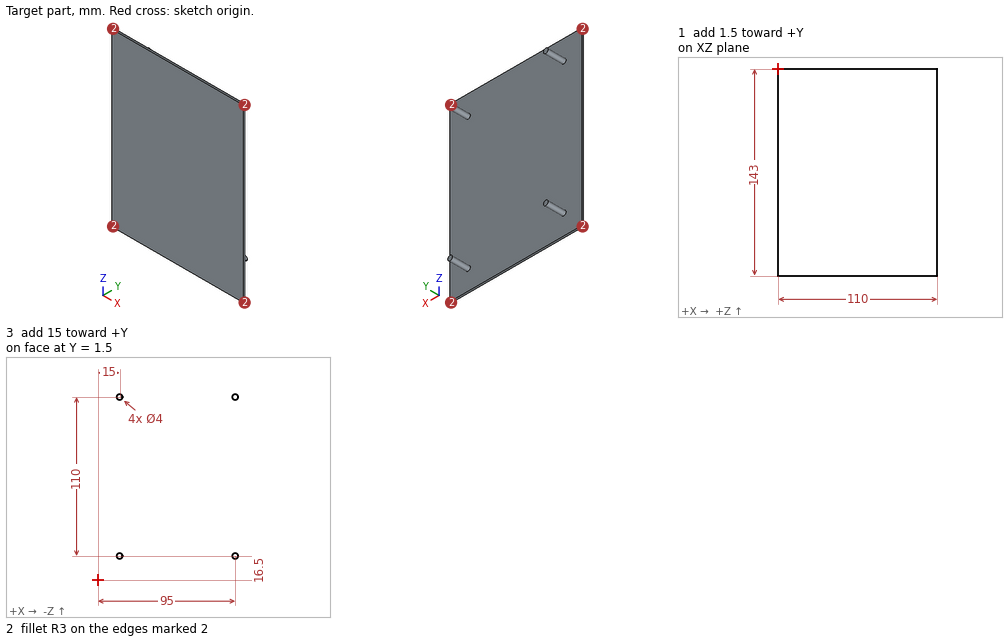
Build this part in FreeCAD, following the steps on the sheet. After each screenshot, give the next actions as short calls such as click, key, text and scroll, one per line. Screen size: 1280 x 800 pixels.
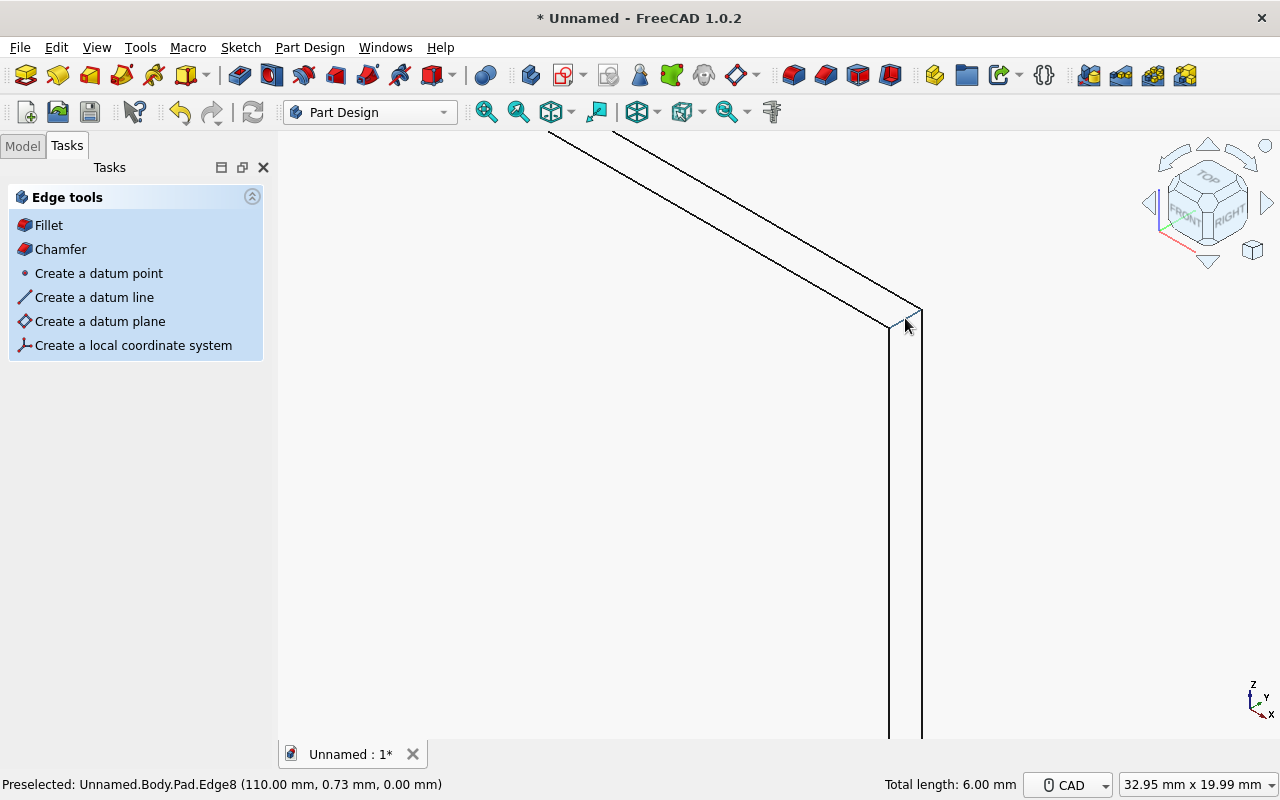
key(v)
key(1)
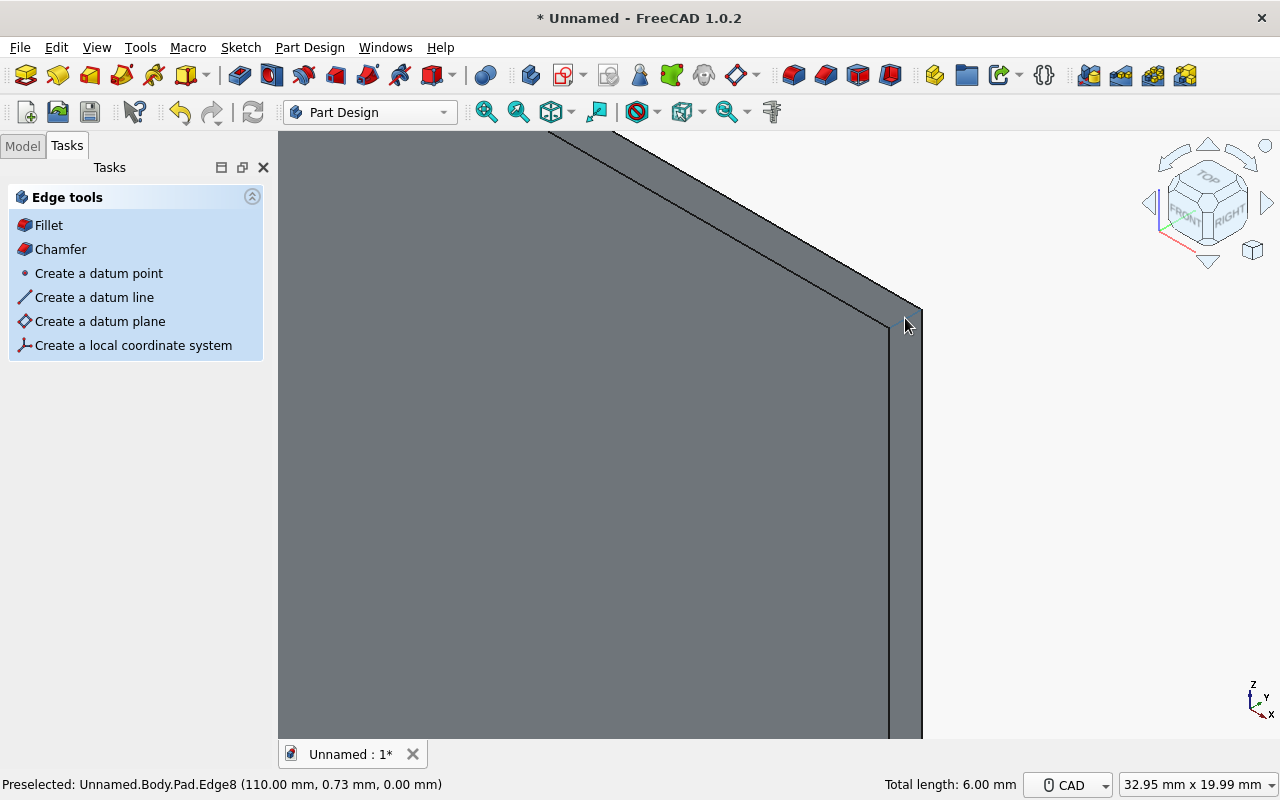
click(794, 76)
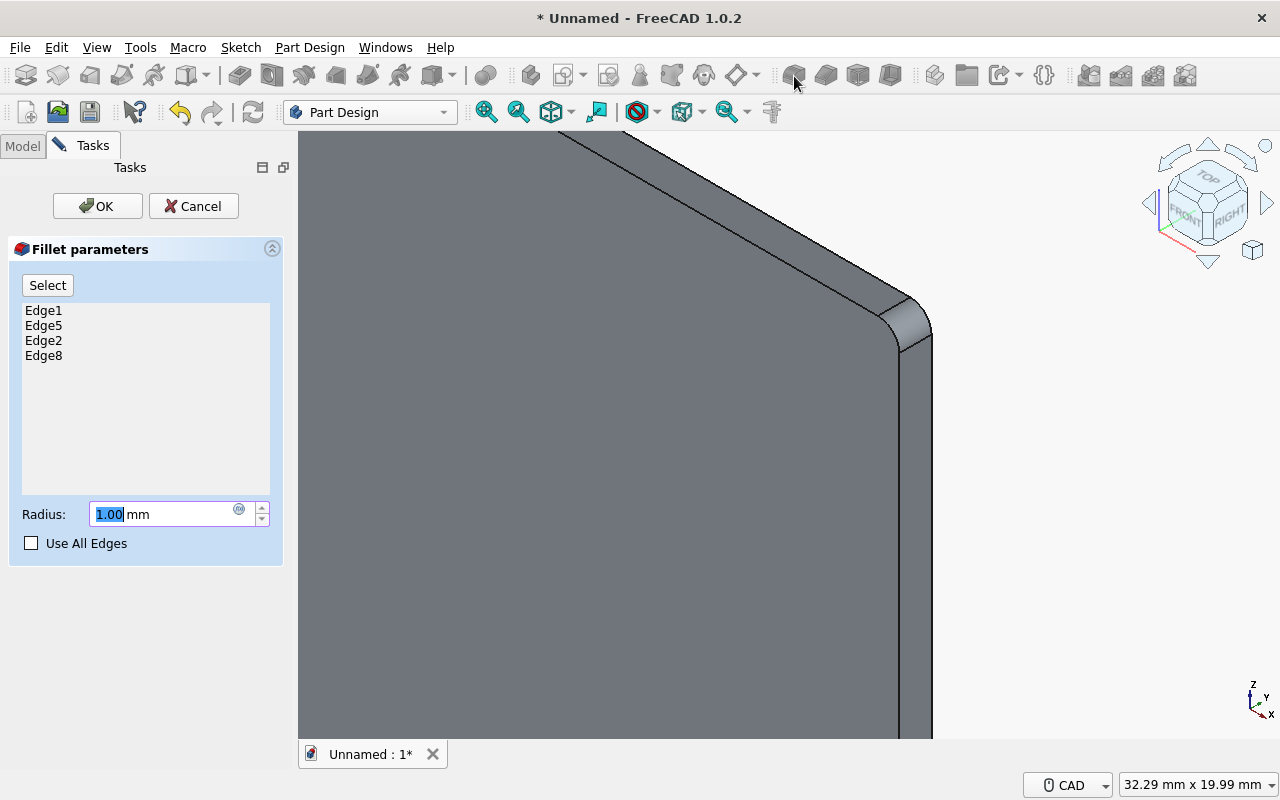
text(3)
key(Tab)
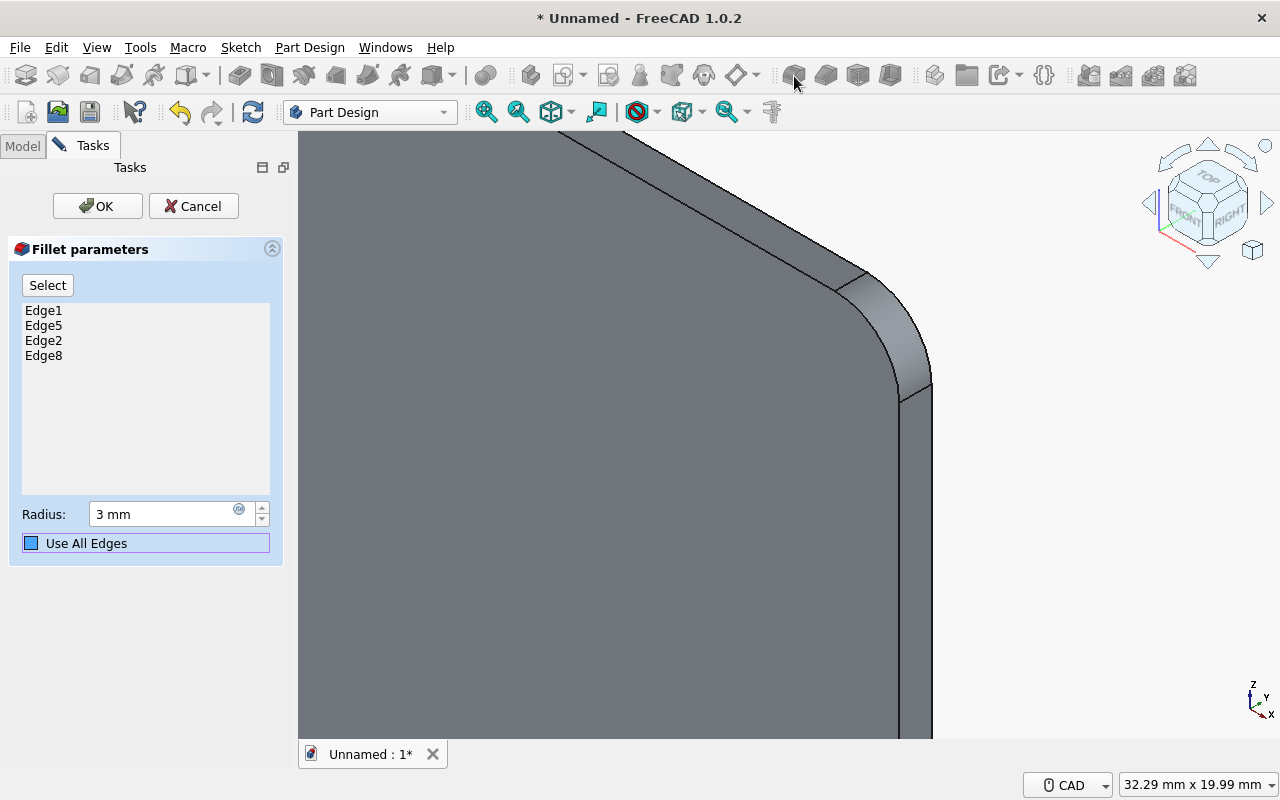
click(98, 206)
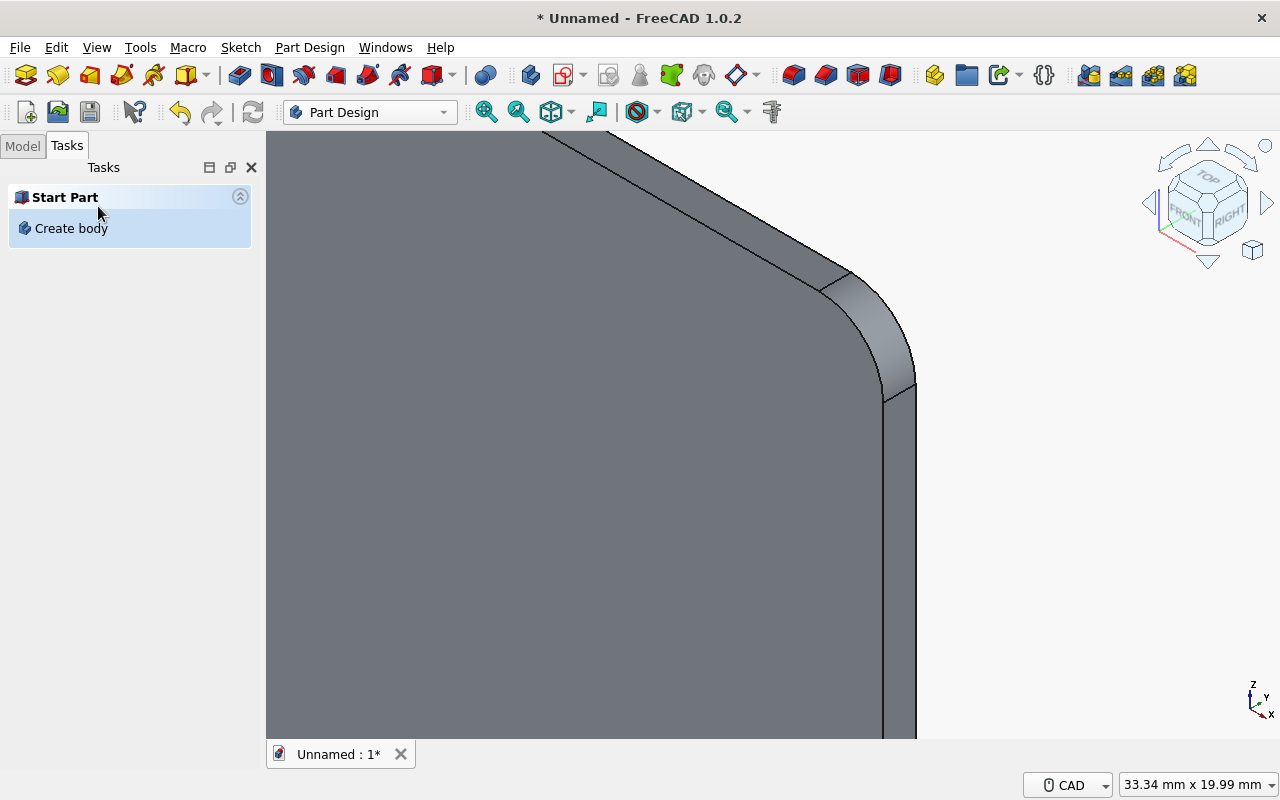
click(488, 112)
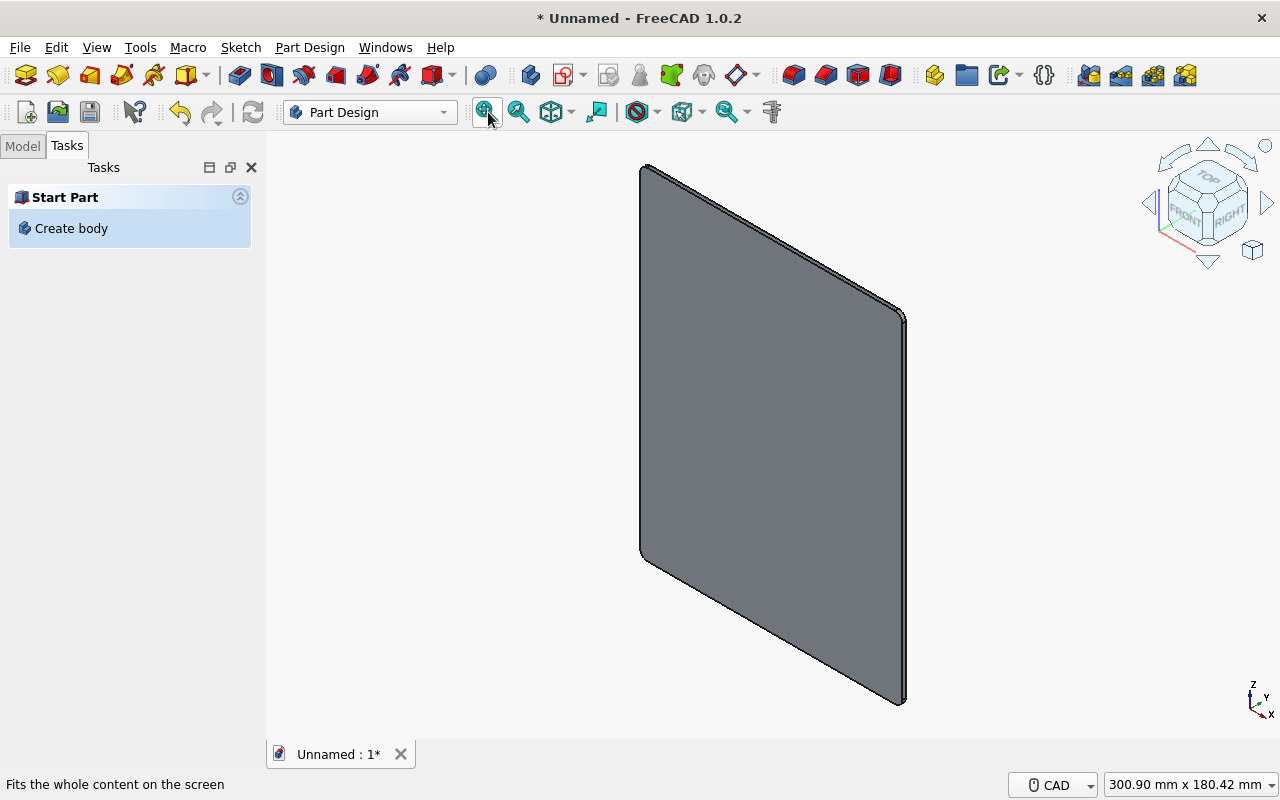
key(4)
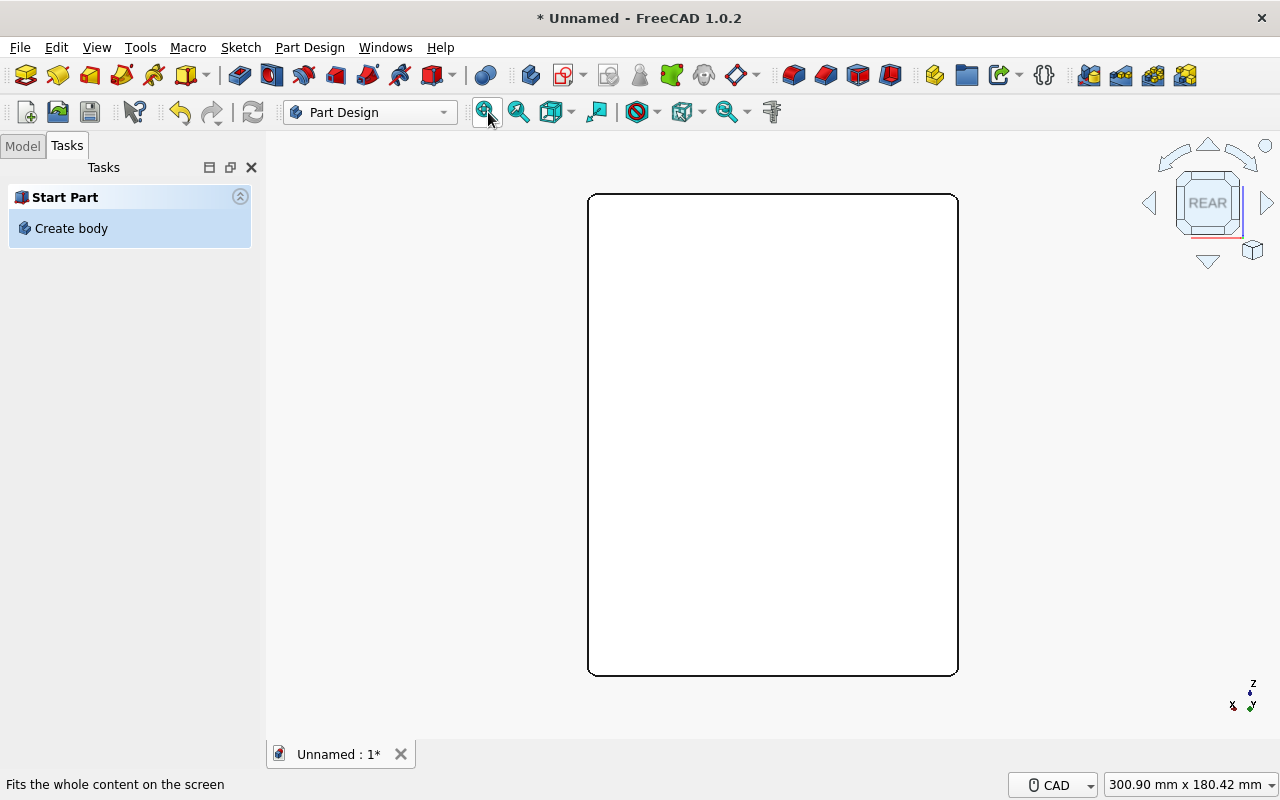
click(773, 434)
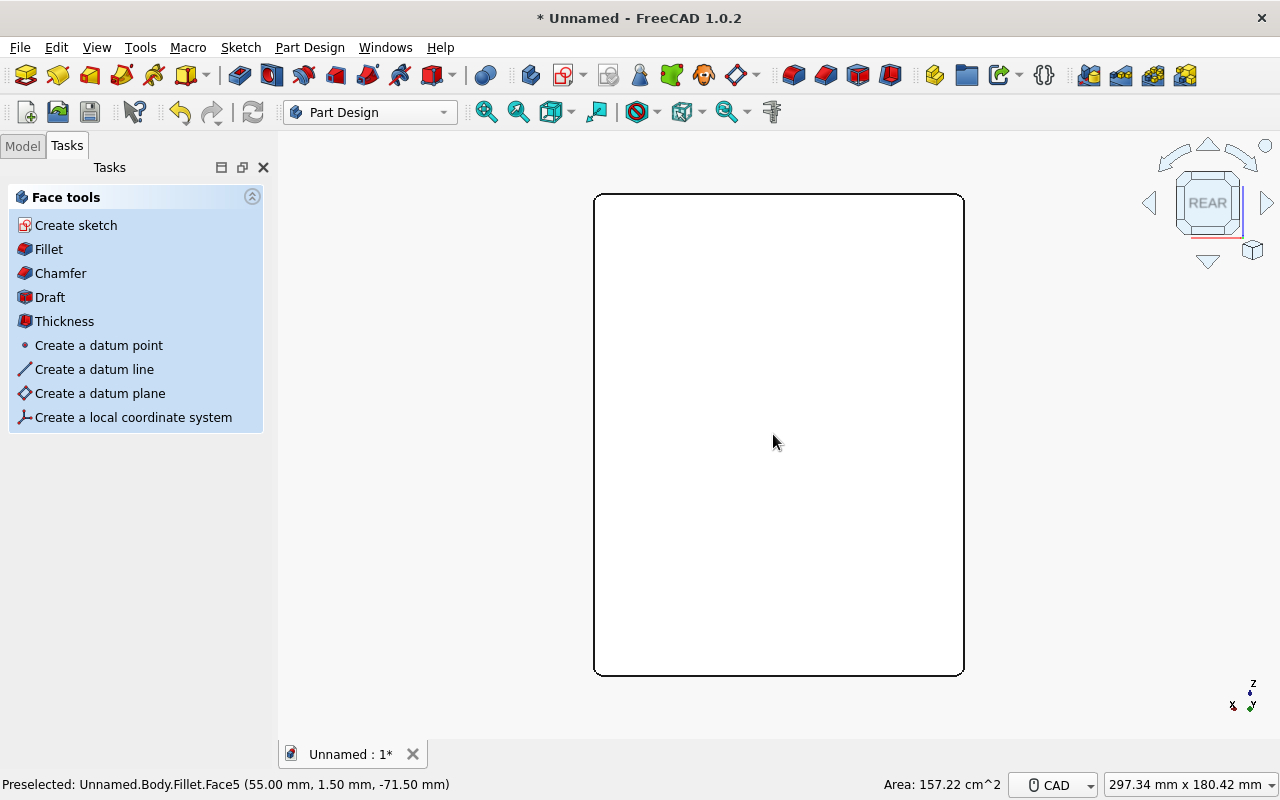
click(564, 76)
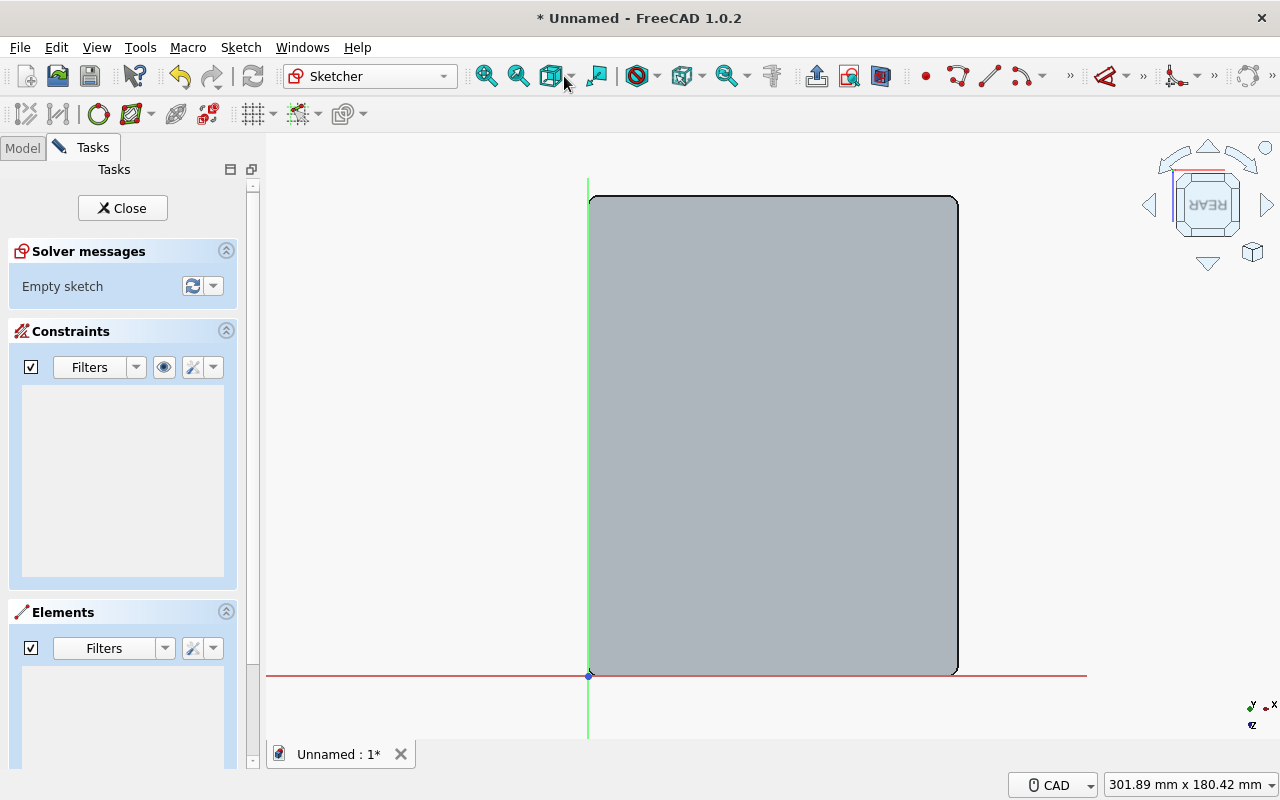
key(g)
key(c)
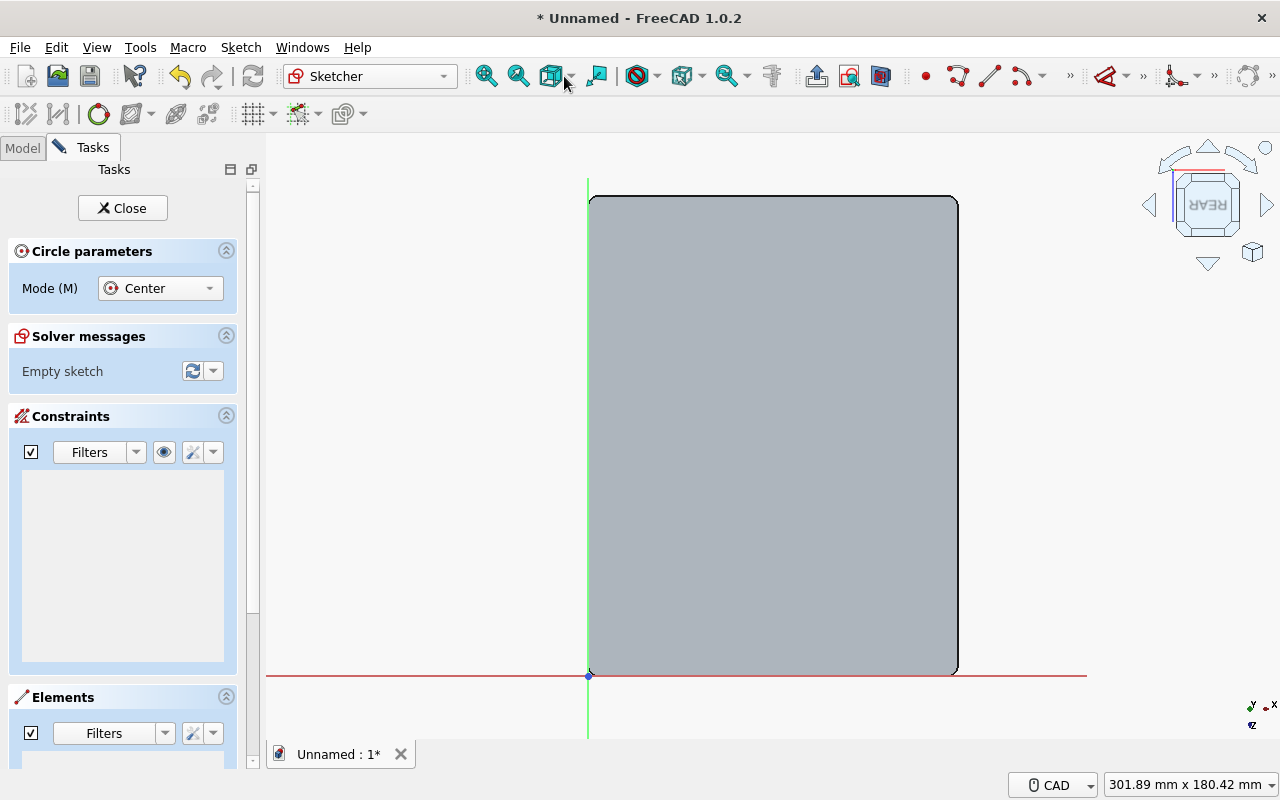
scroll(639, 251, up, 7)